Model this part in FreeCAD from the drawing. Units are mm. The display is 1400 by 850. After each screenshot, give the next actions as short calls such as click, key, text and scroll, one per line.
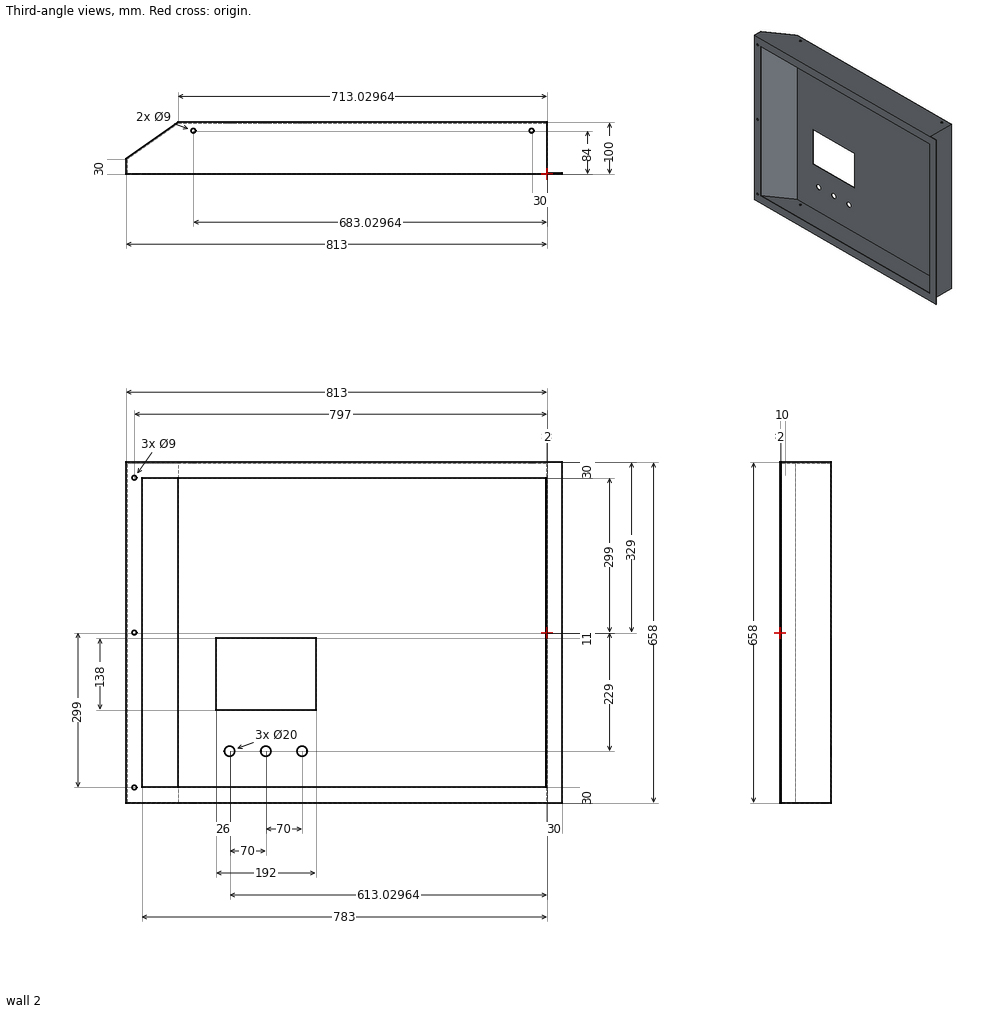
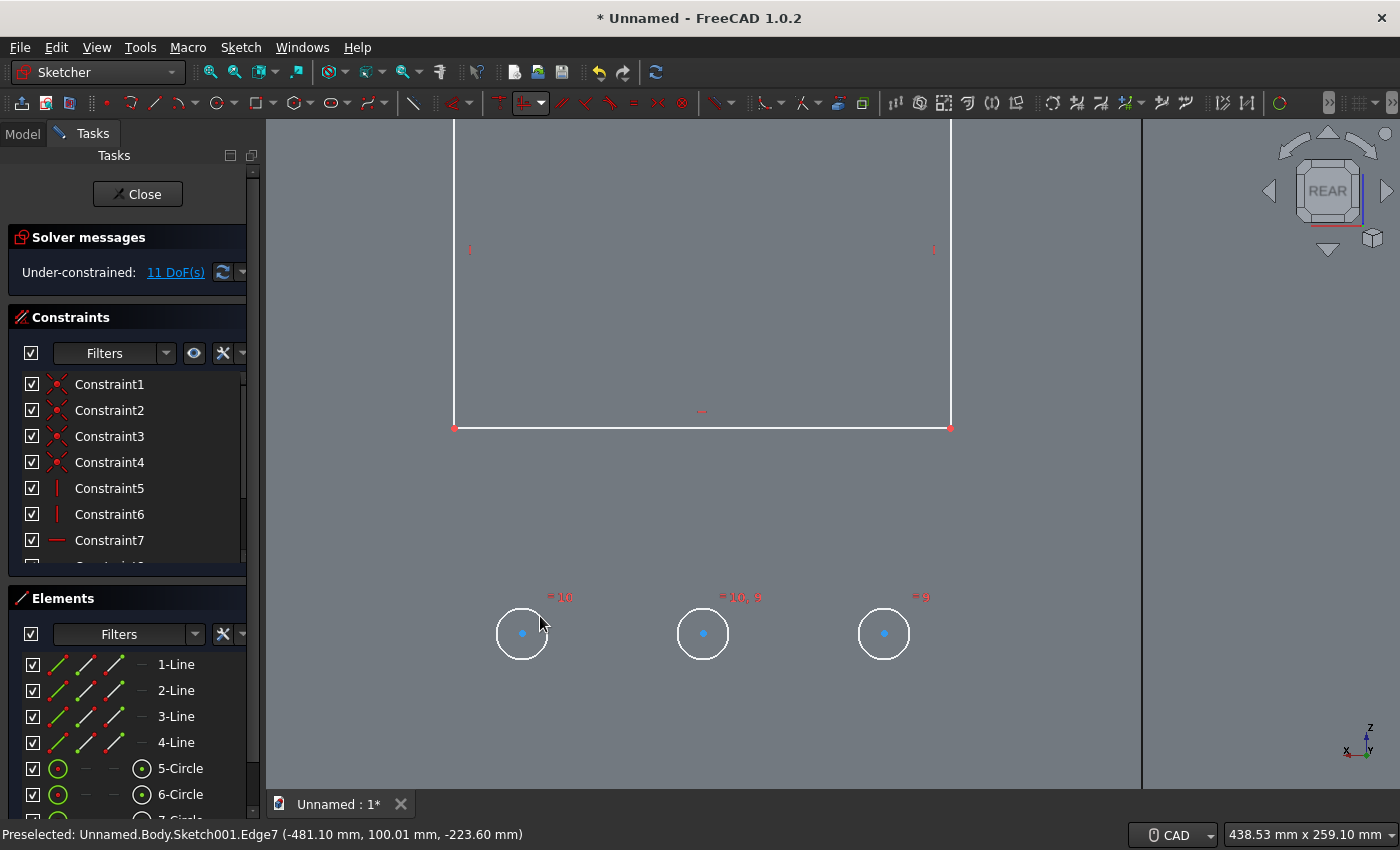
click(884, 634)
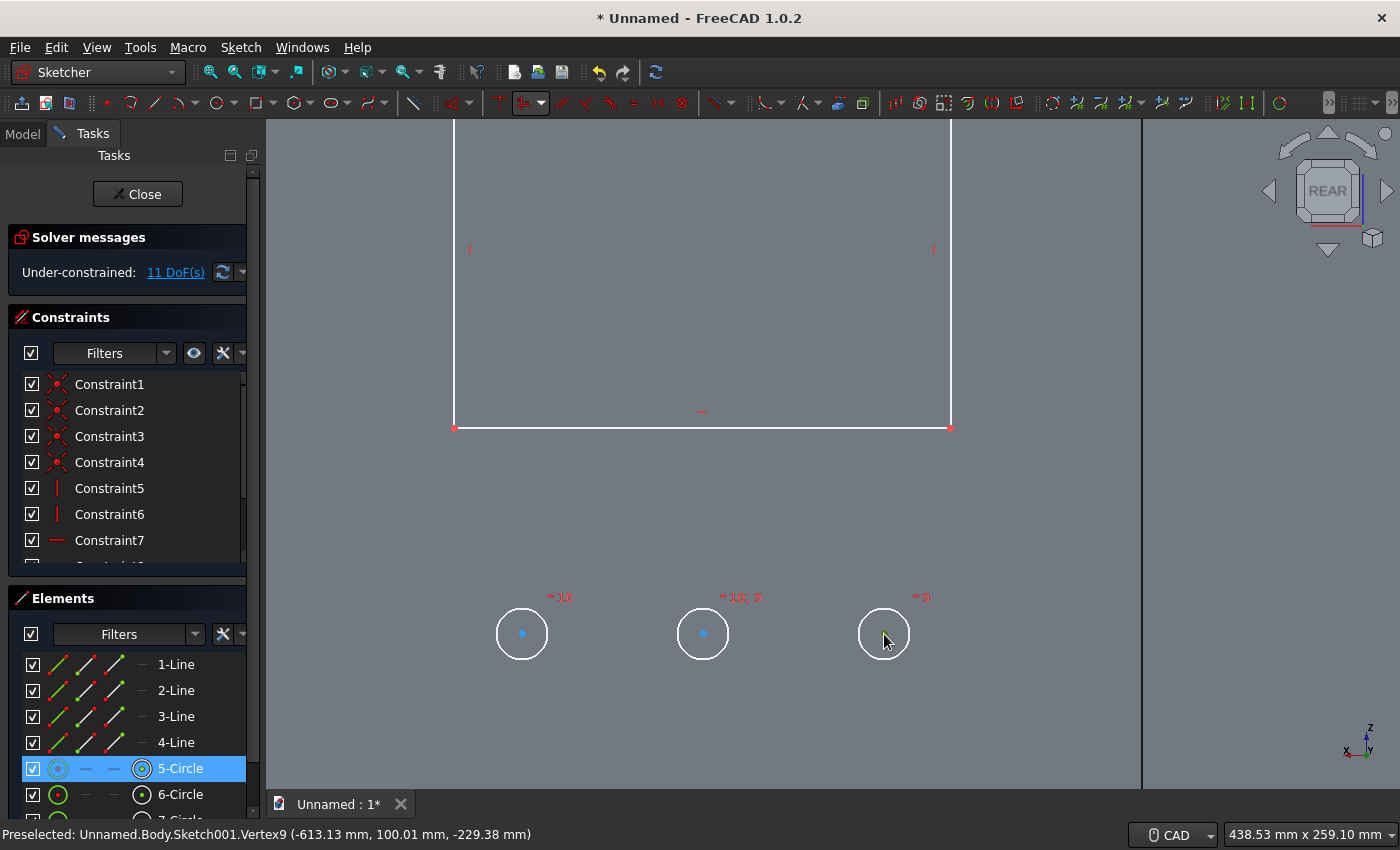
click(703, 634)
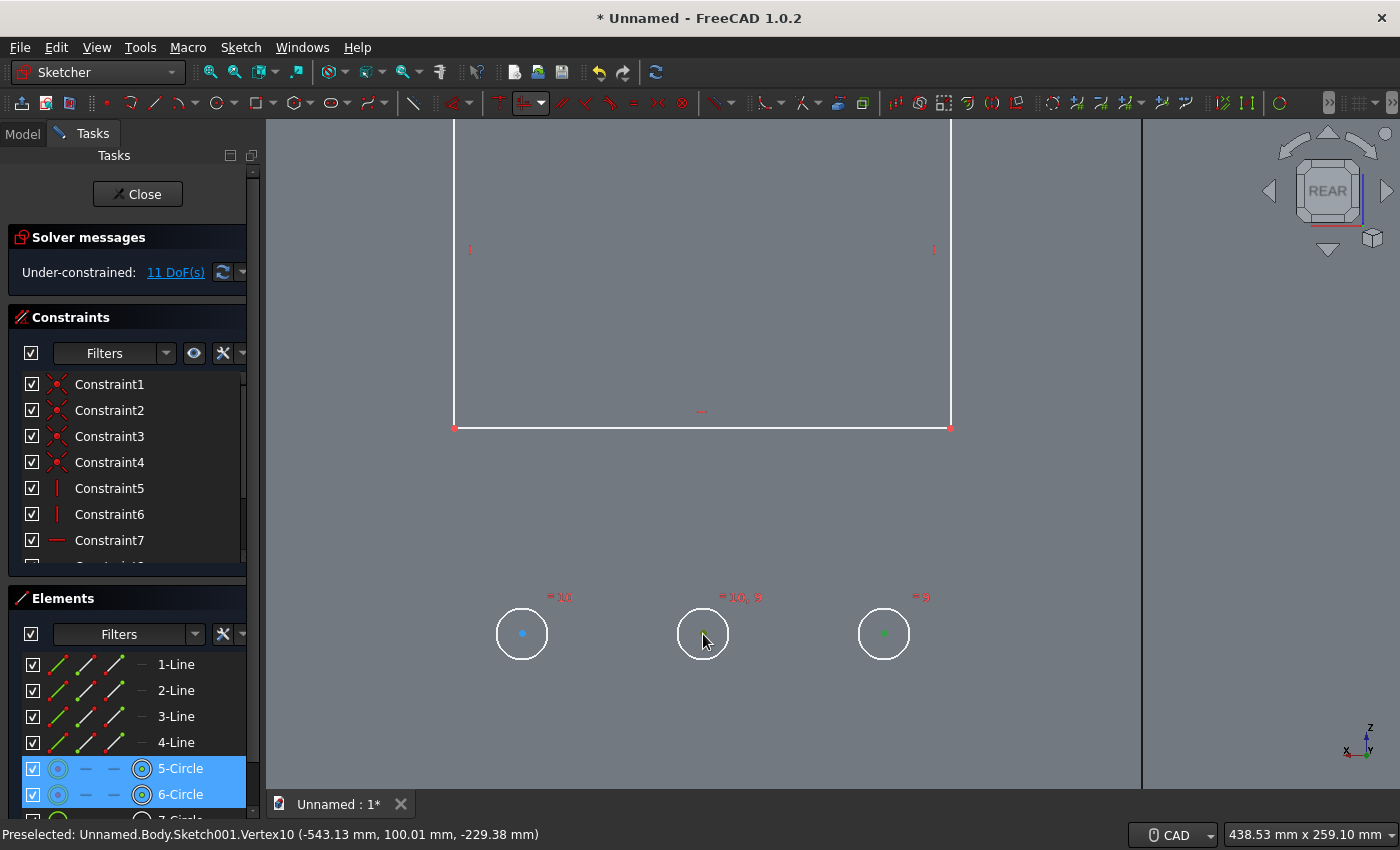
key(h)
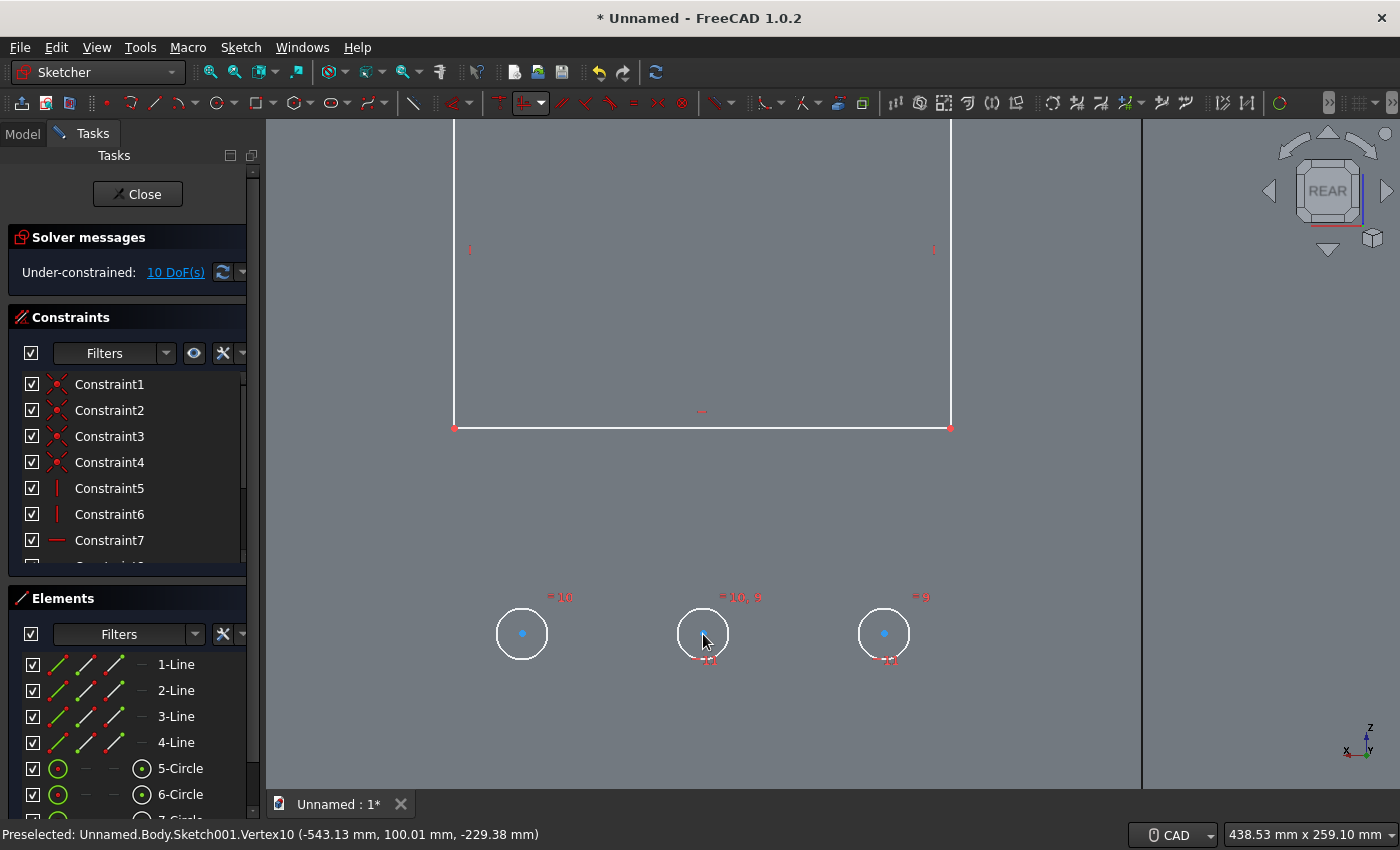
click(703, 634)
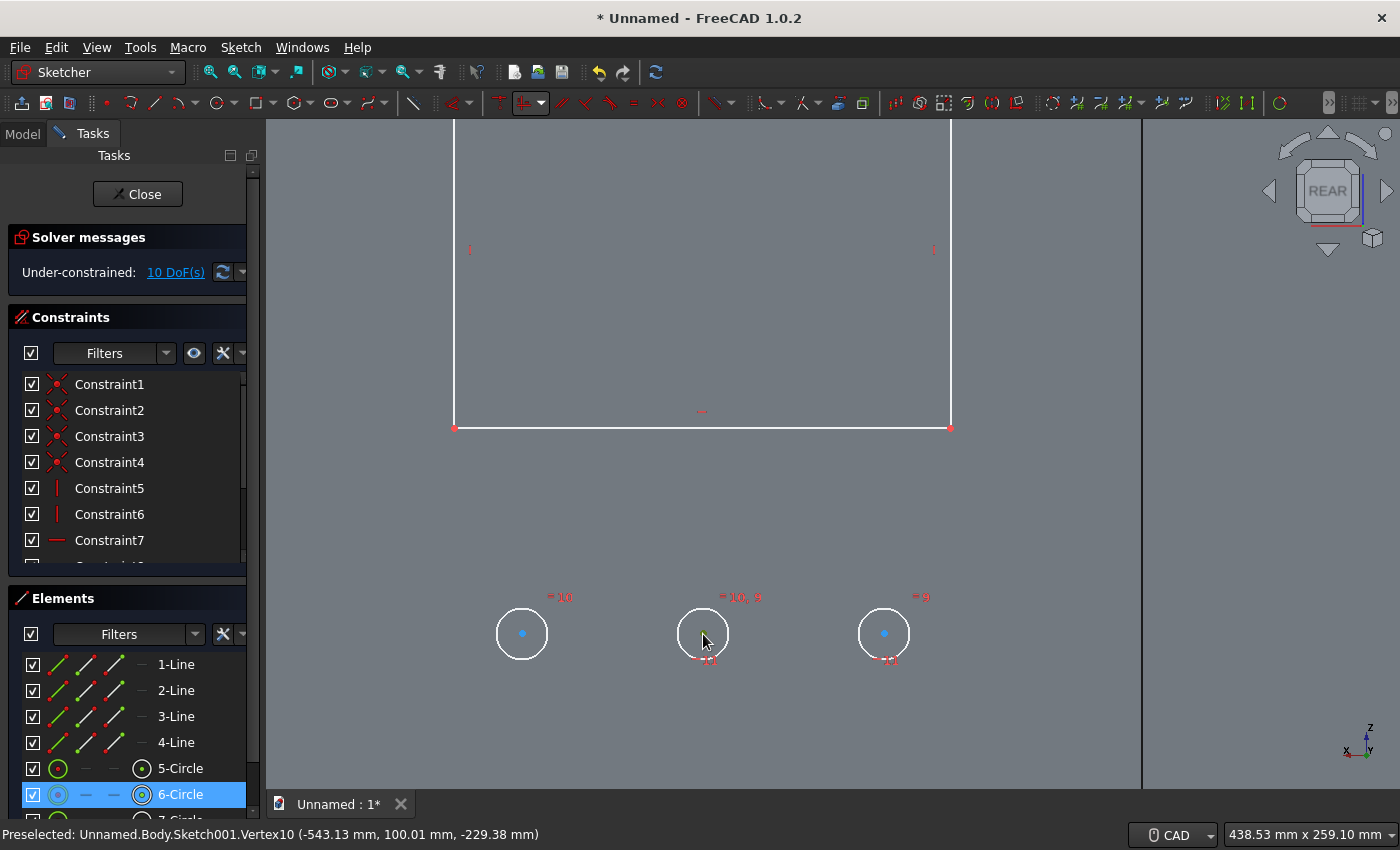
click(522, 634)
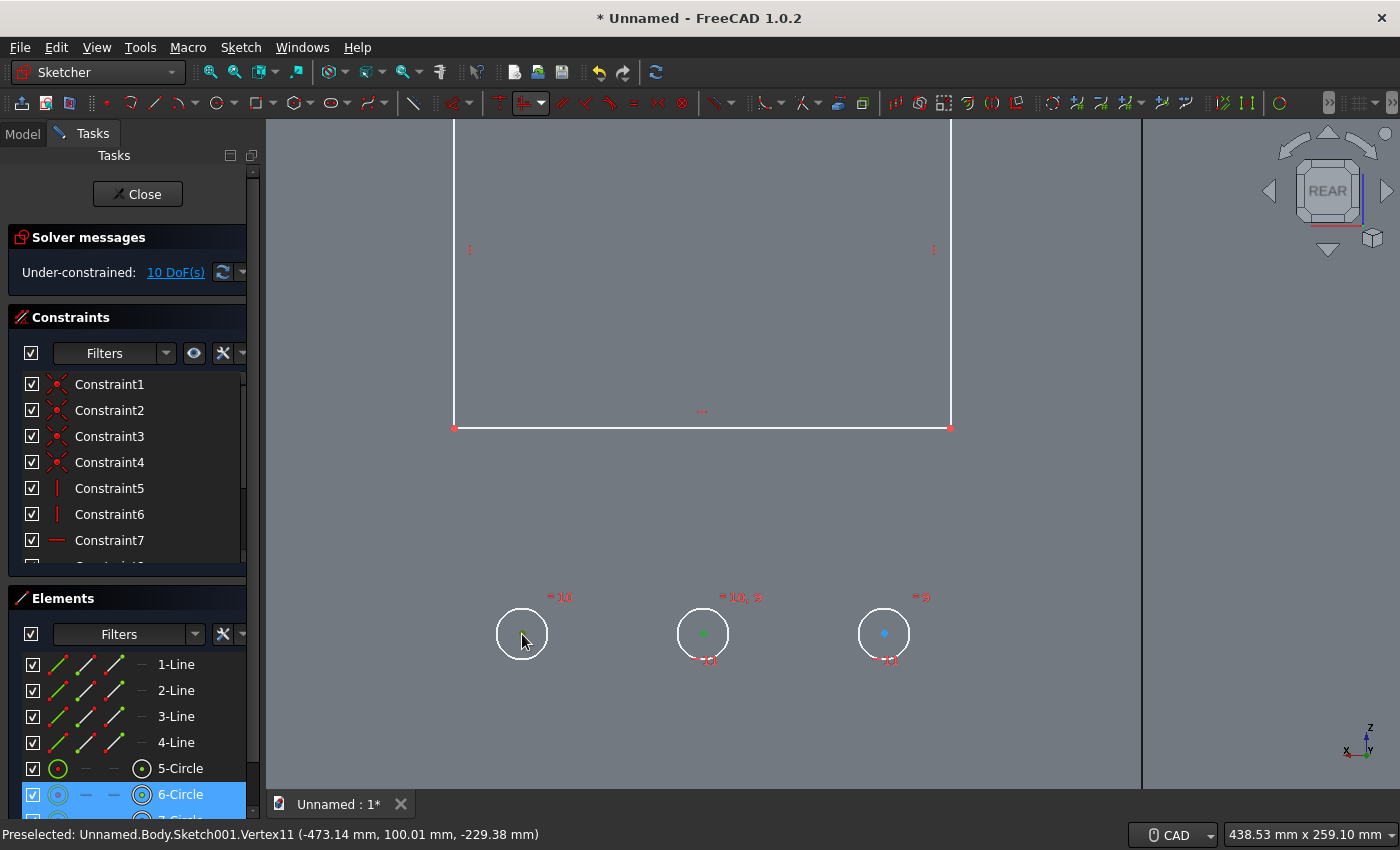
key(h)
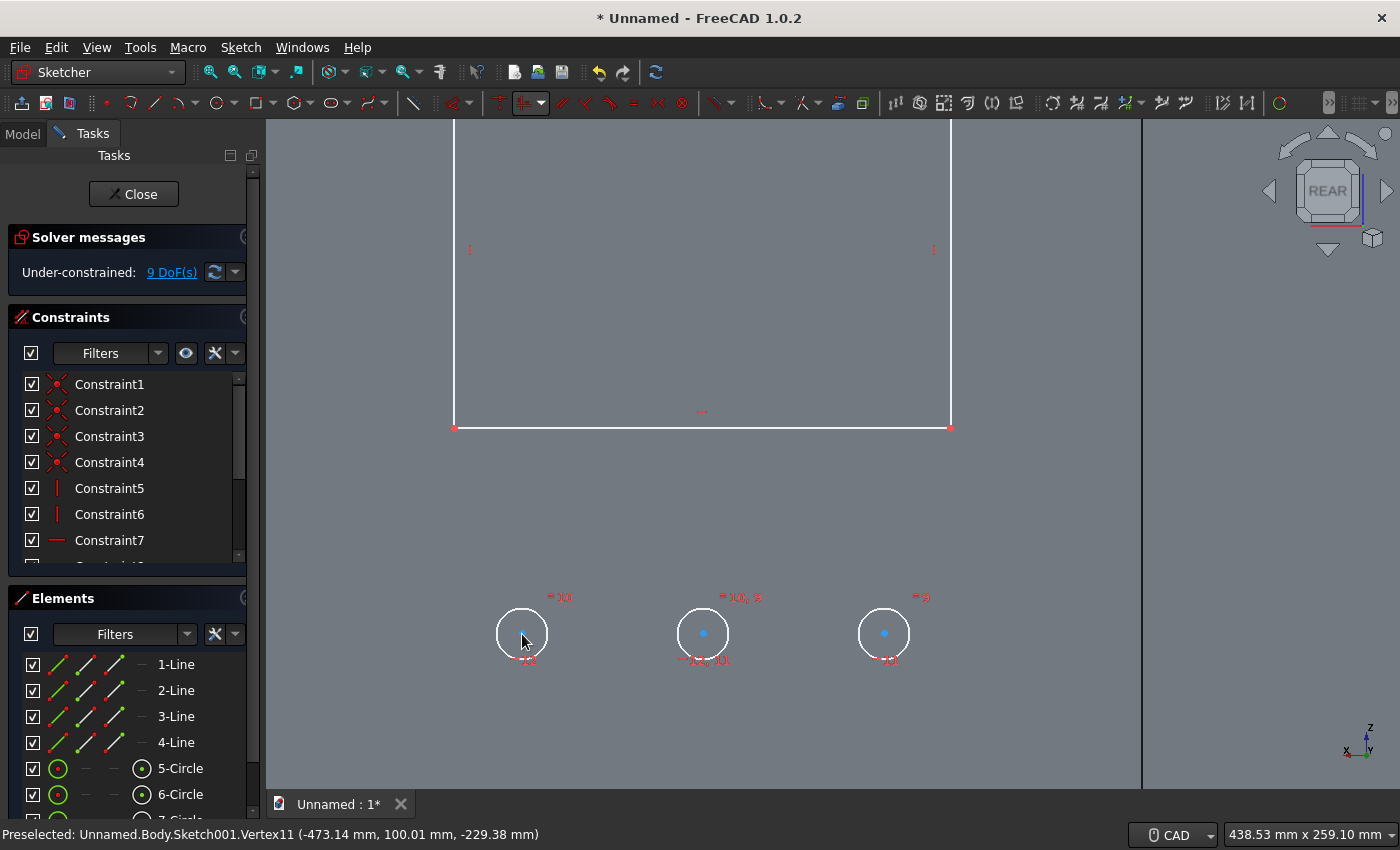
click(452, 104)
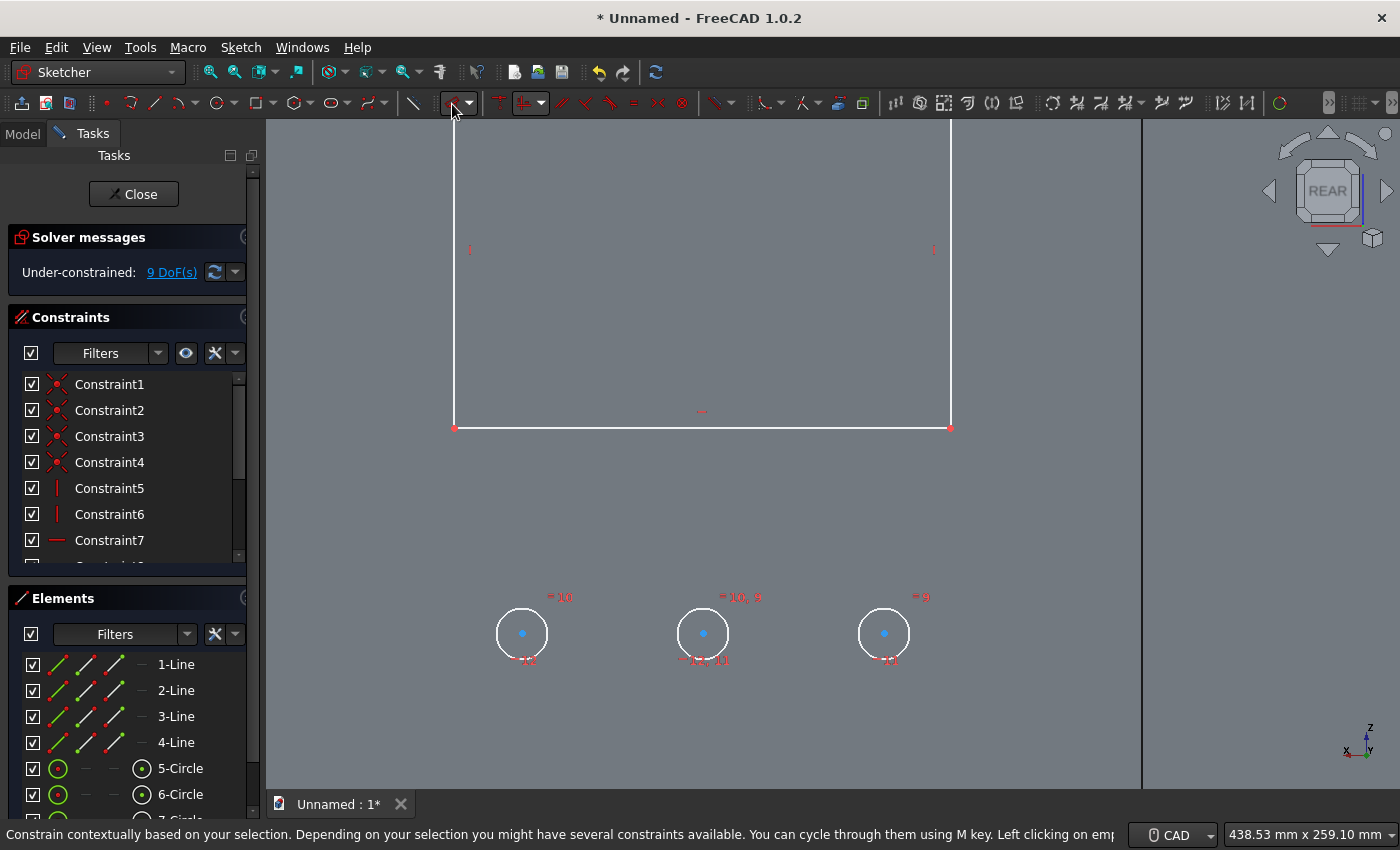
click(902, 616)
click(925, 593)